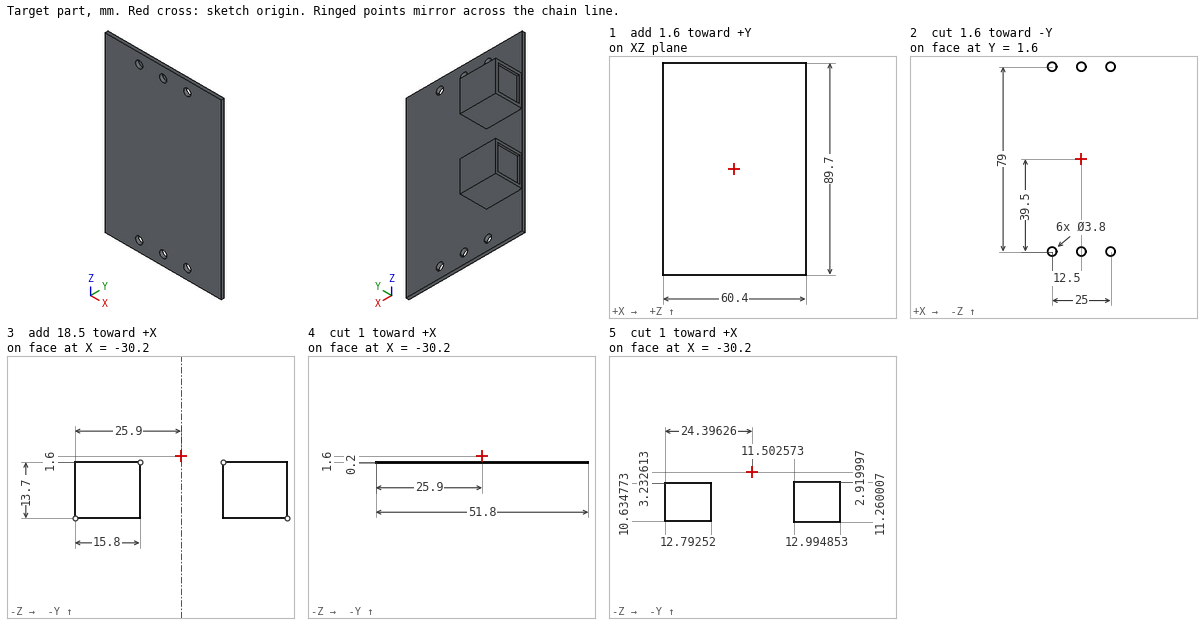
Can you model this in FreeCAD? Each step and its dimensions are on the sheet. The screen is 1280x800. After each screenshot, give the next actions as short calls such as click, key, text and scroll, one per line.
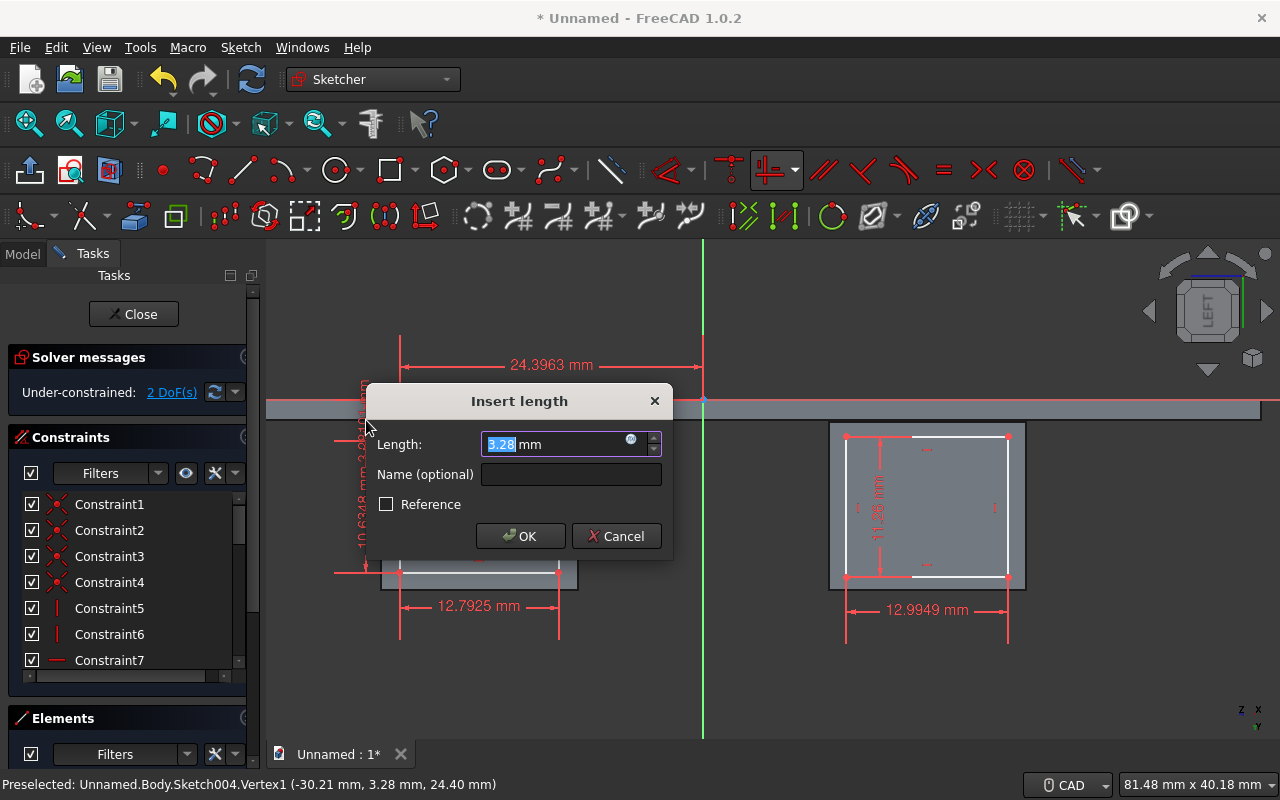
text(3.232613)
key(Return)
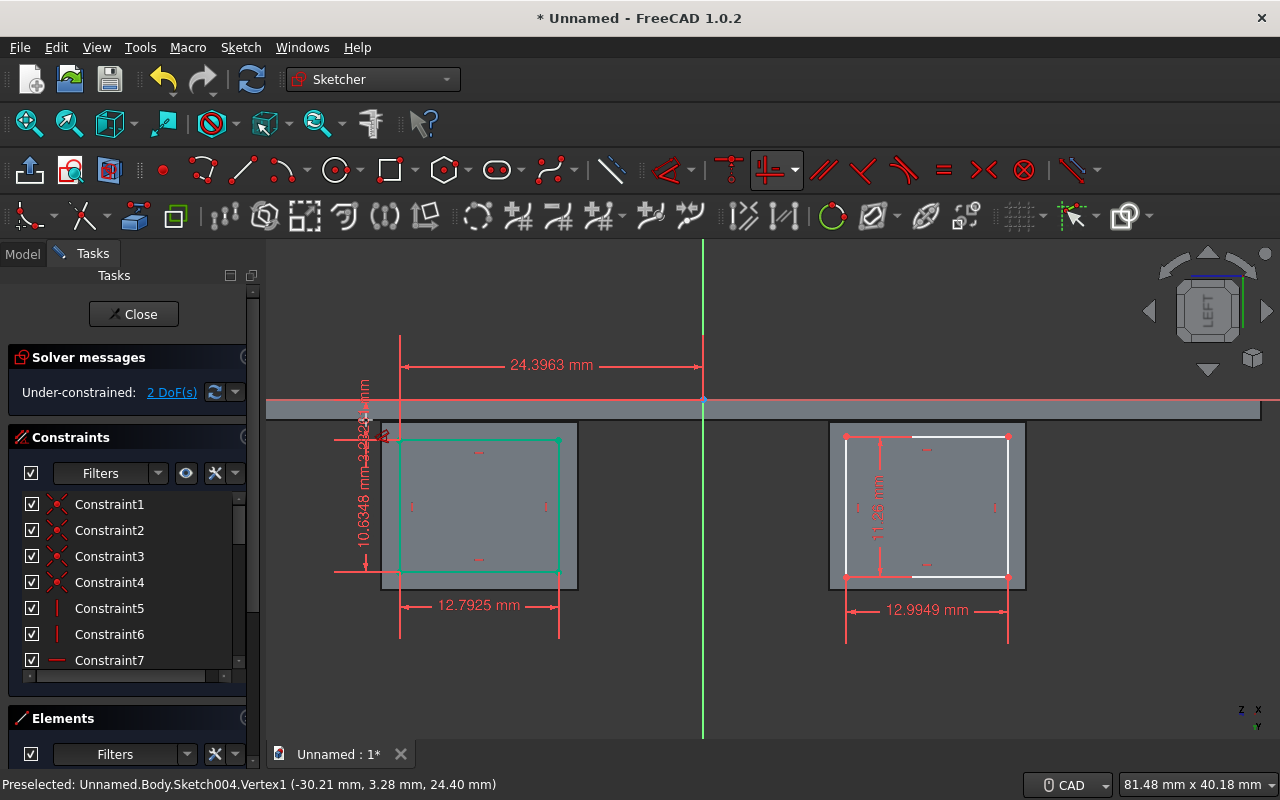
click(846, 437)
click(880, 418)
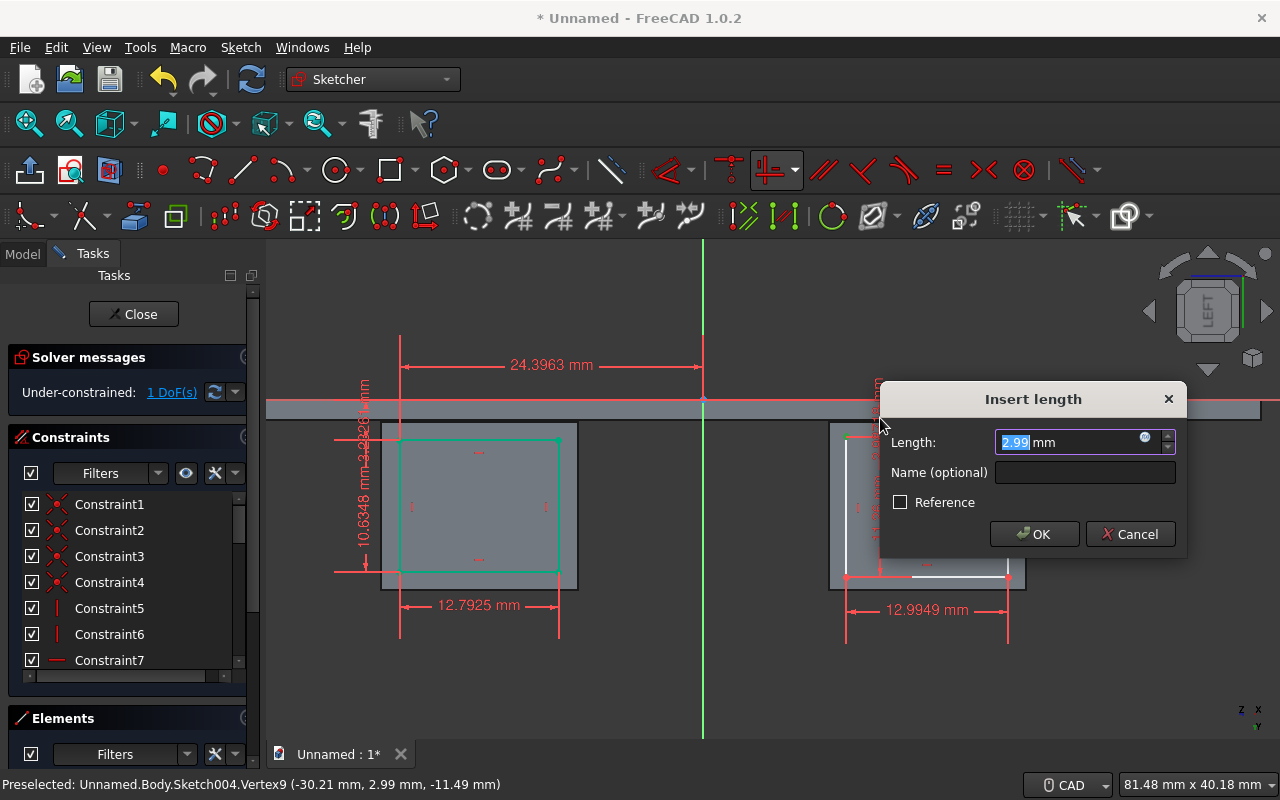
text(2.919997)
key(Return)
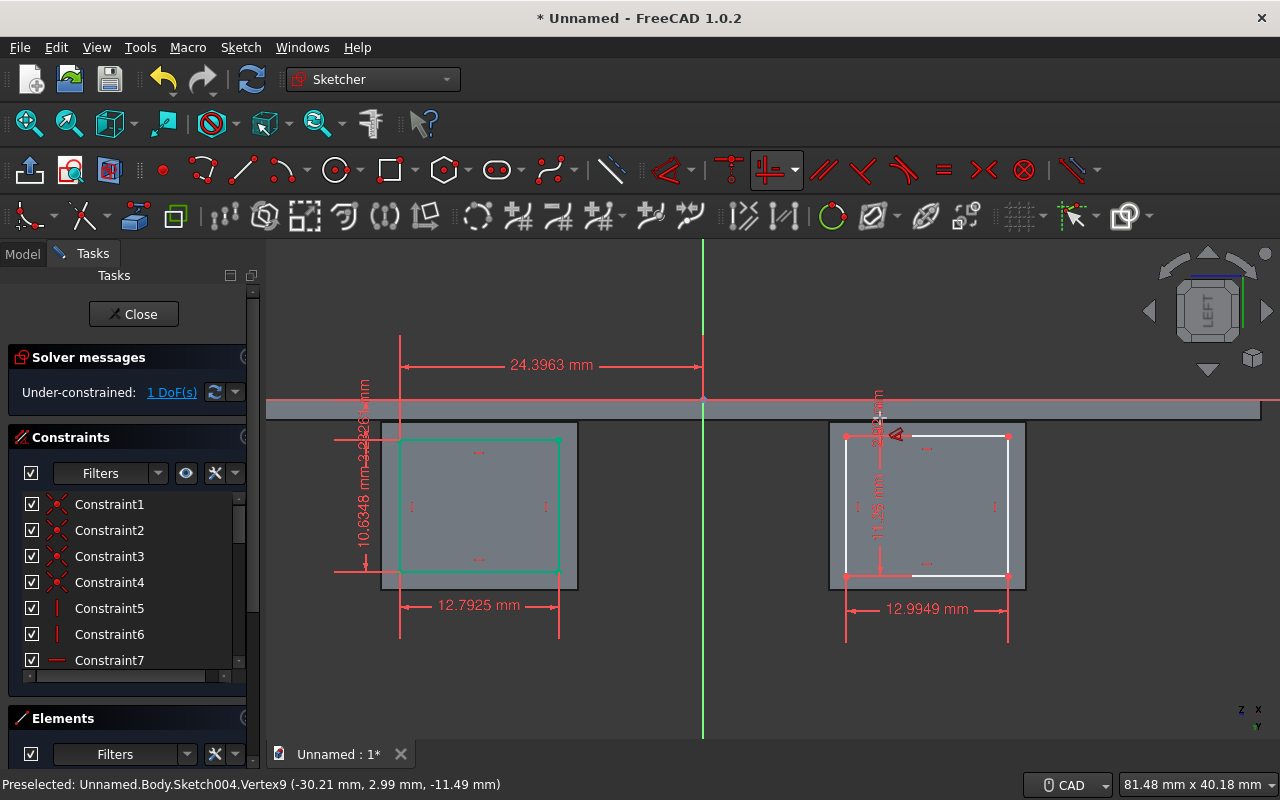
click(846, 436)
click(775, 366)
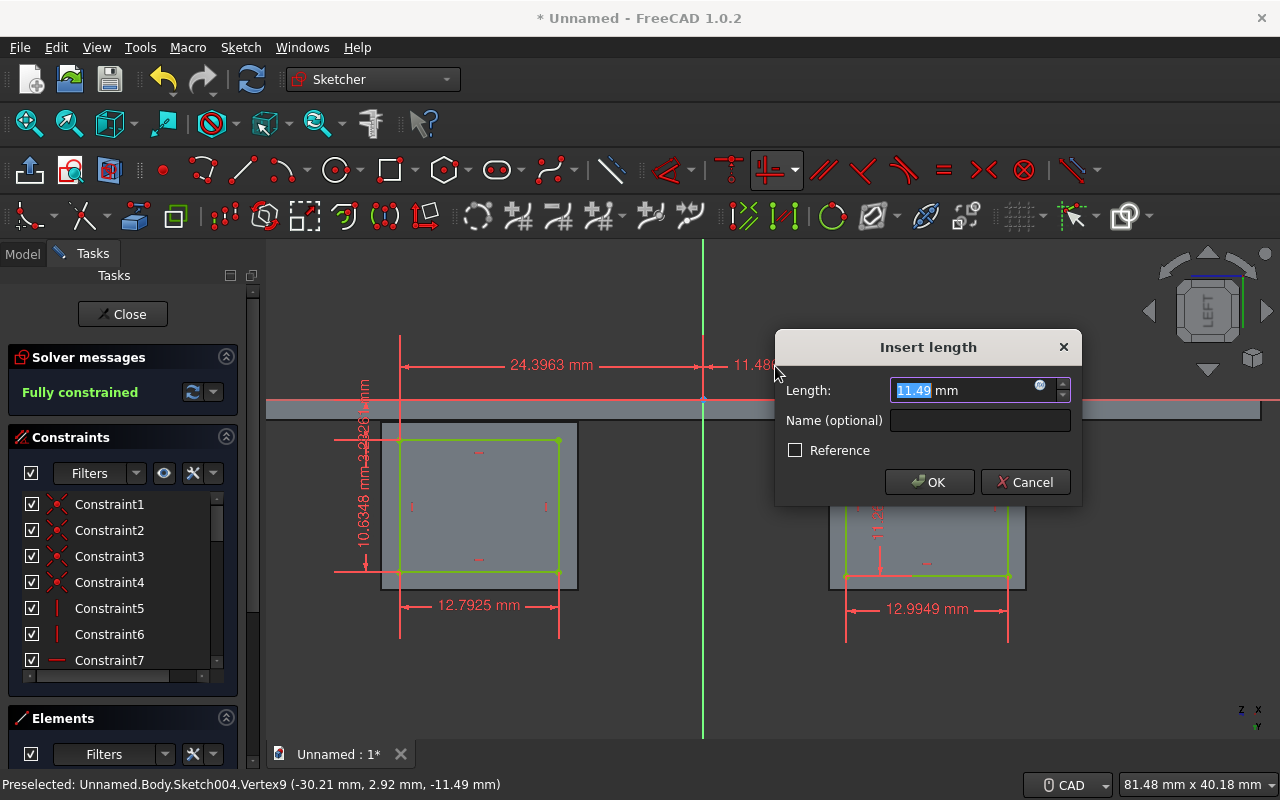
text(11.502573)
key(Return)
key(Escape)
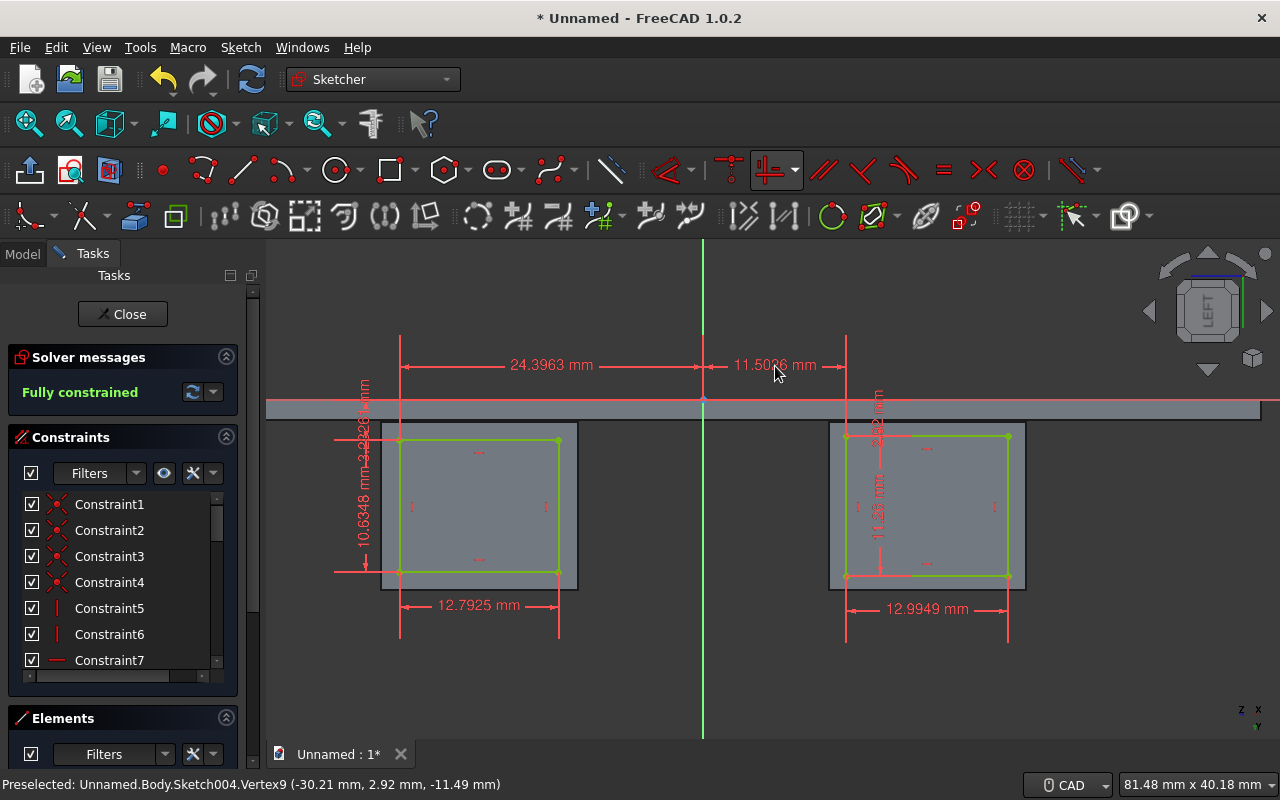
click(123, 314)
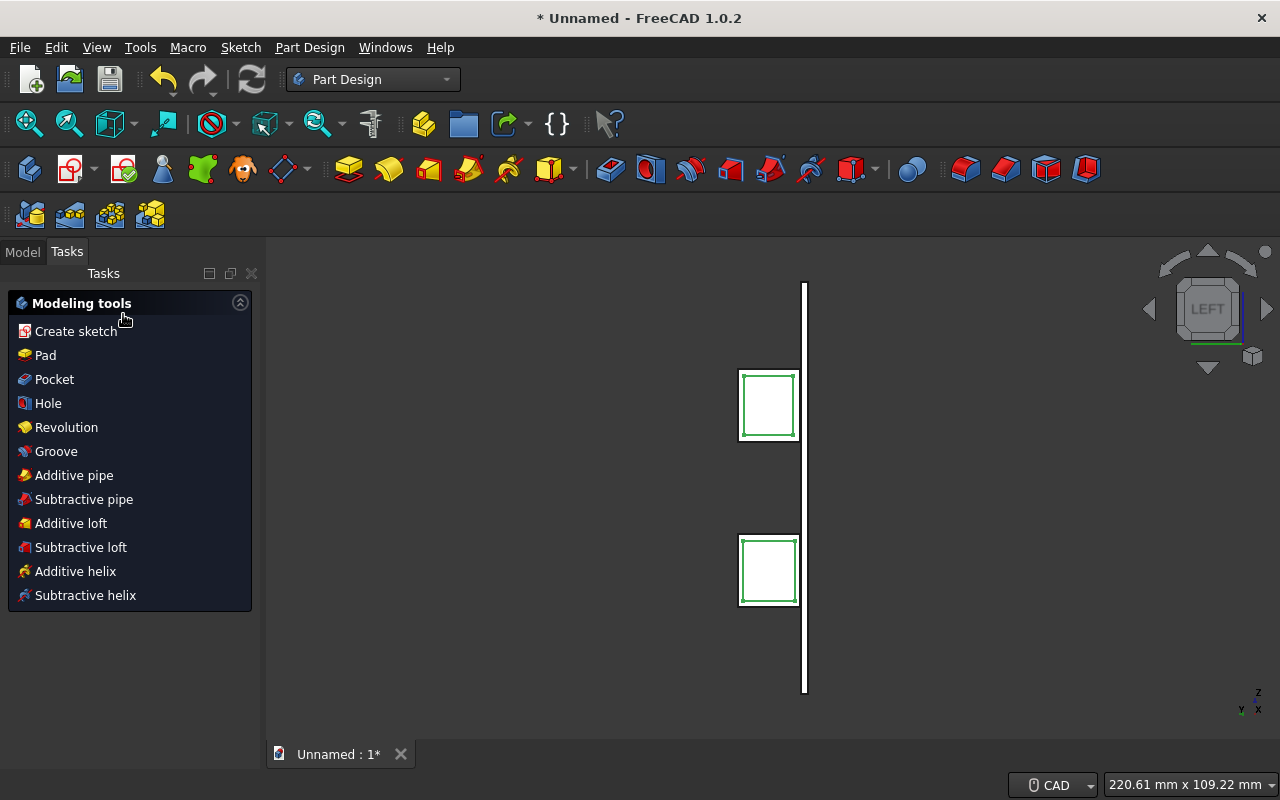
click(612, 170)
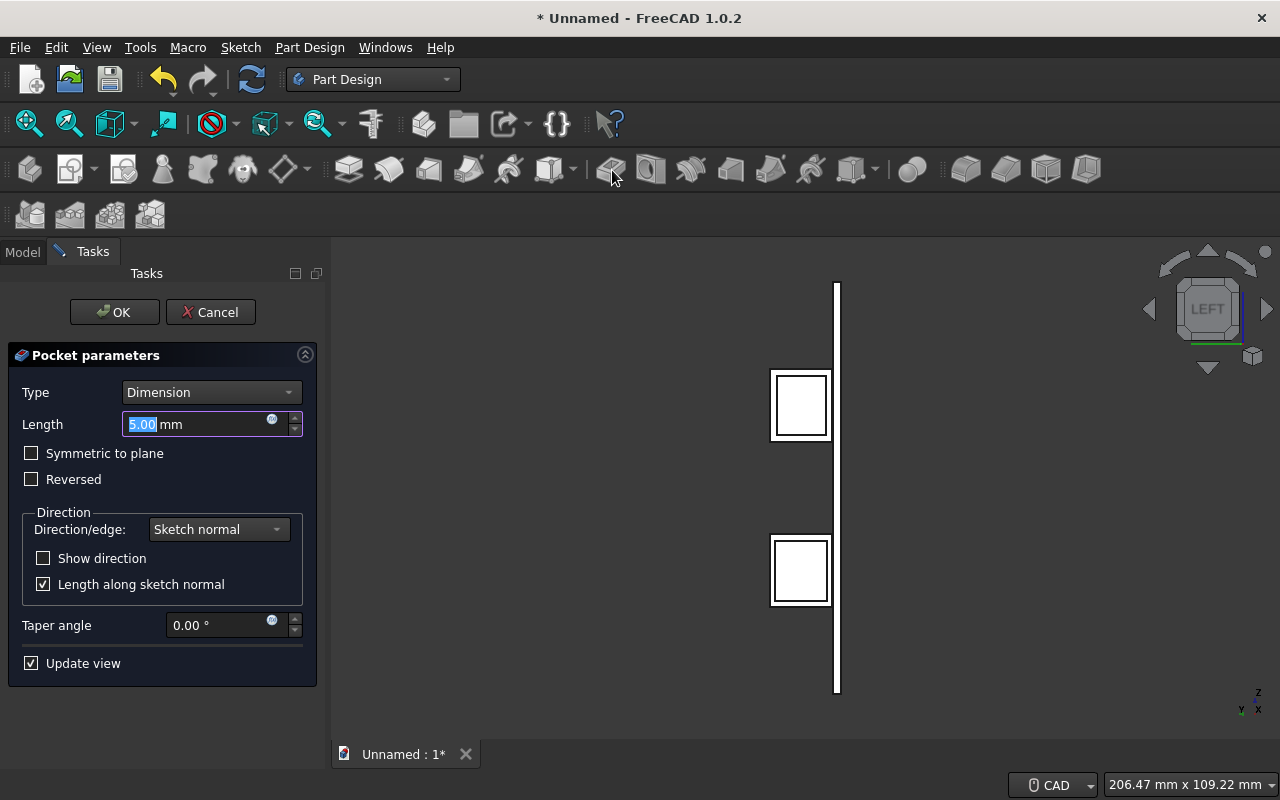
text(1)
key(Tab)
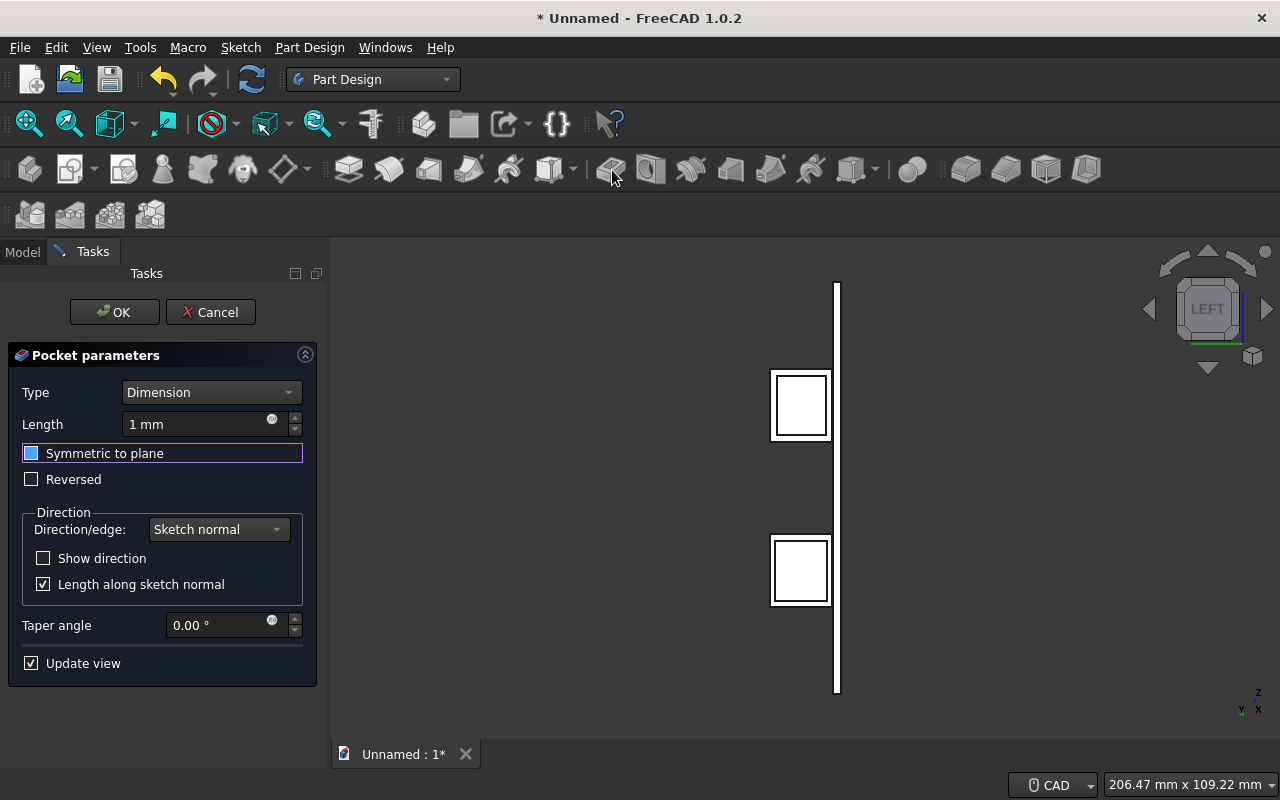
click(115, 312)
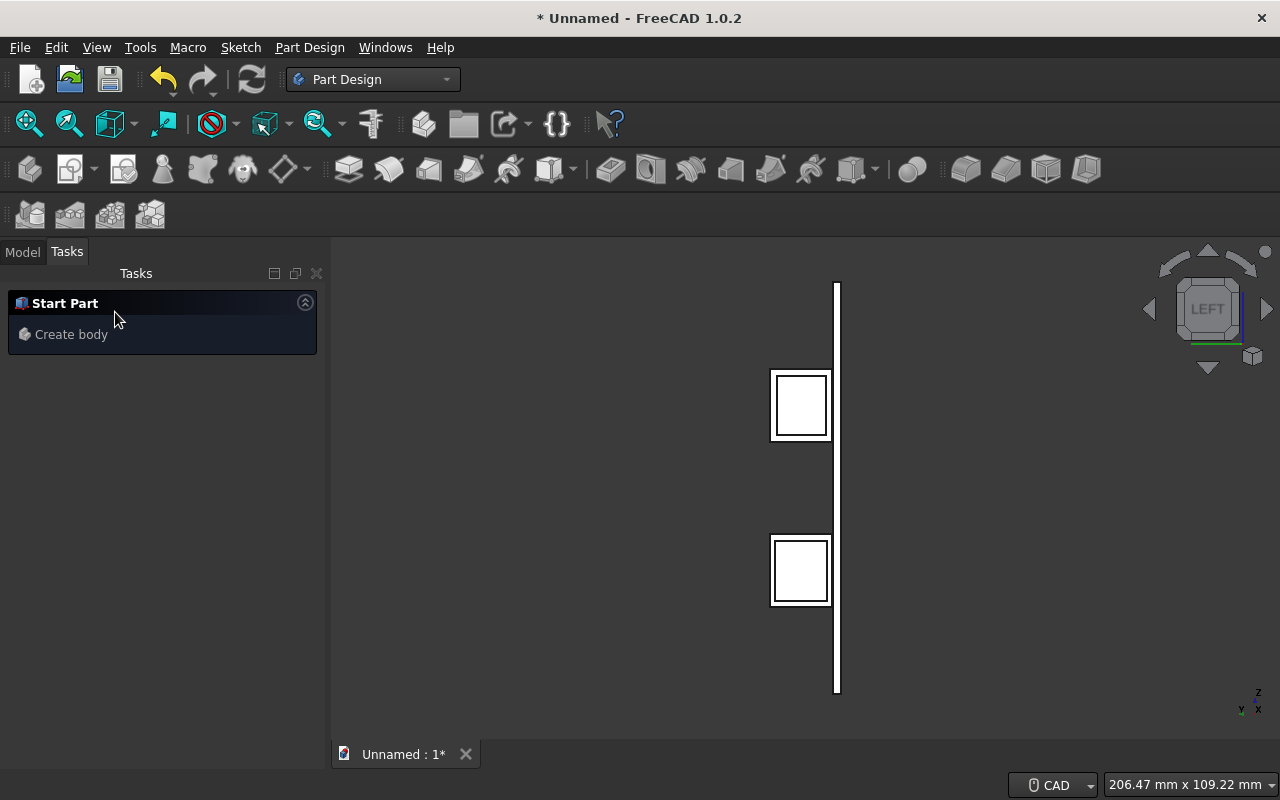
key(0)